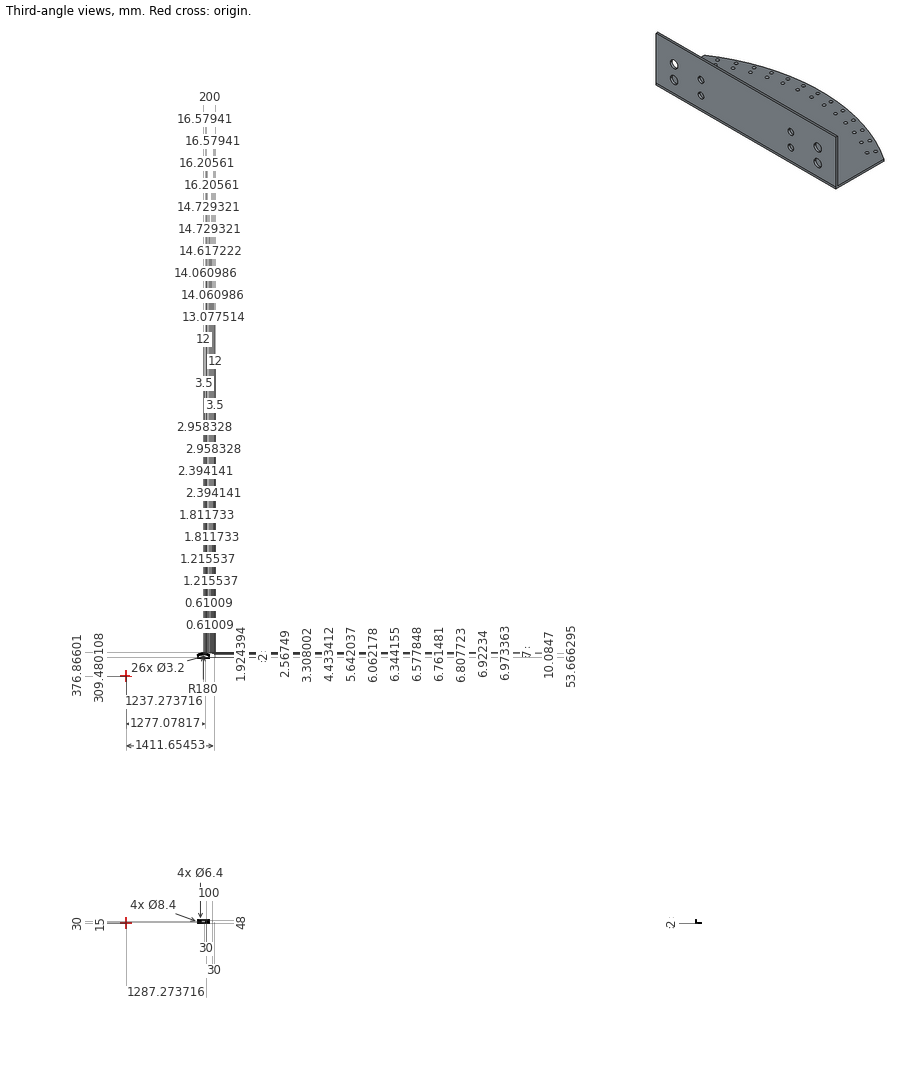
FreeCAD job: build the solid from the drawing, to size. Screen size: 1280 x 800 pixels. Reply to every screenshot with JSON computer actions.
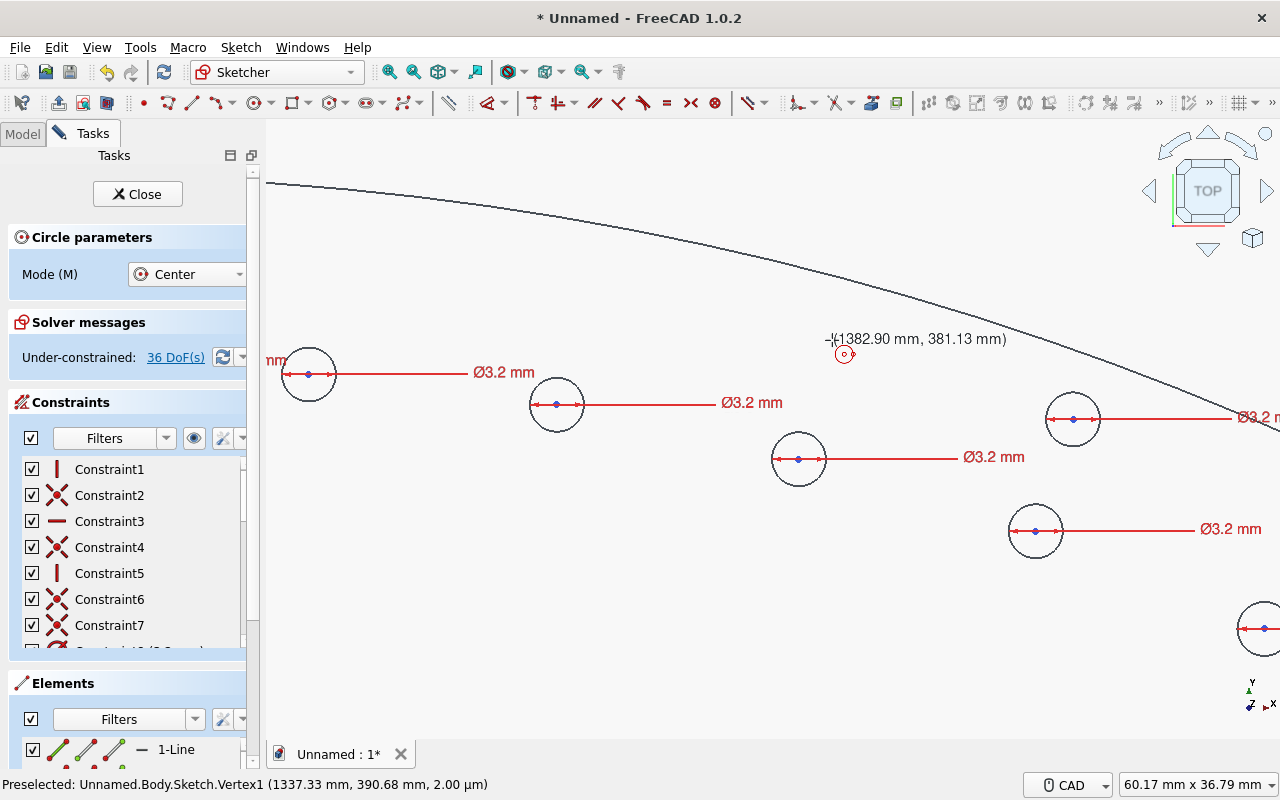
{"action": "scroll", "coordinate": [832, 340], "scroll_direction": "down", "scroll_amount": 9}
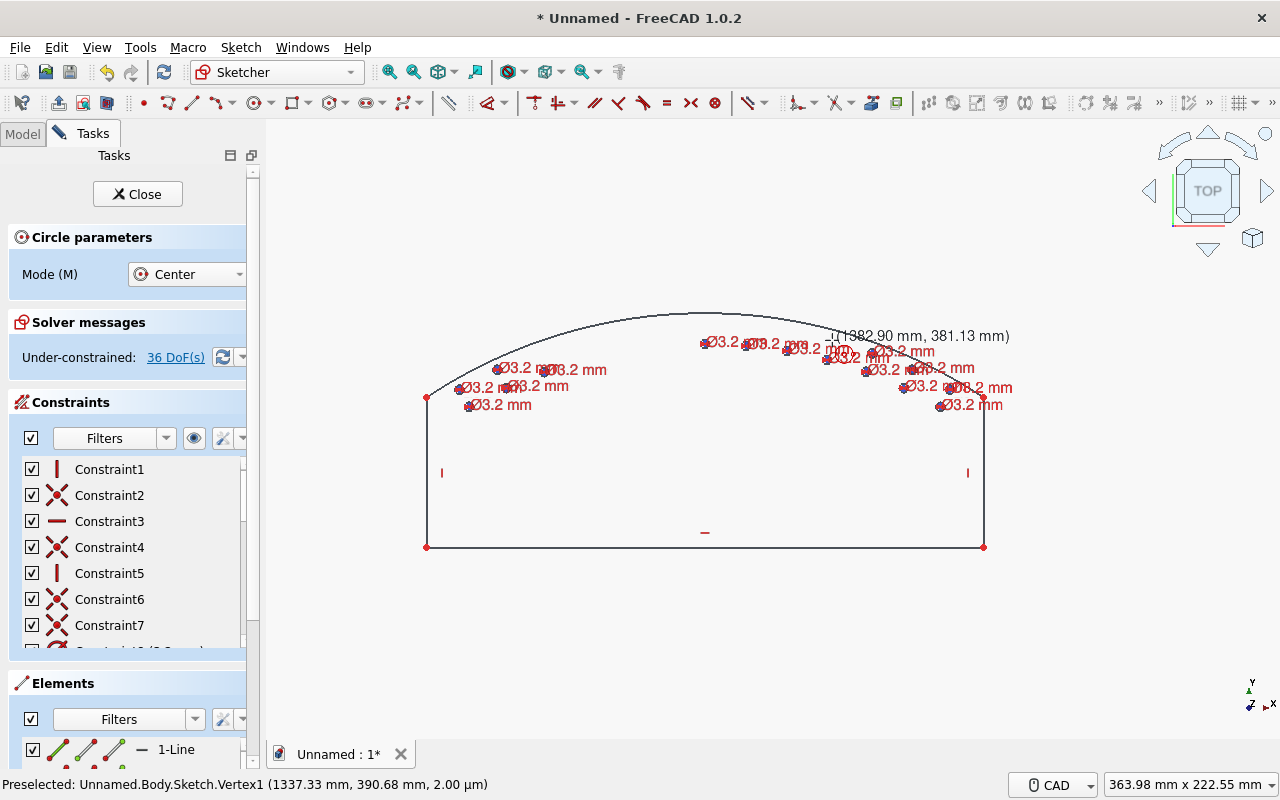
{"action": "scroll", "coordinate": [832, 340], "scroll_direction": "up", "scroll_amount": 2}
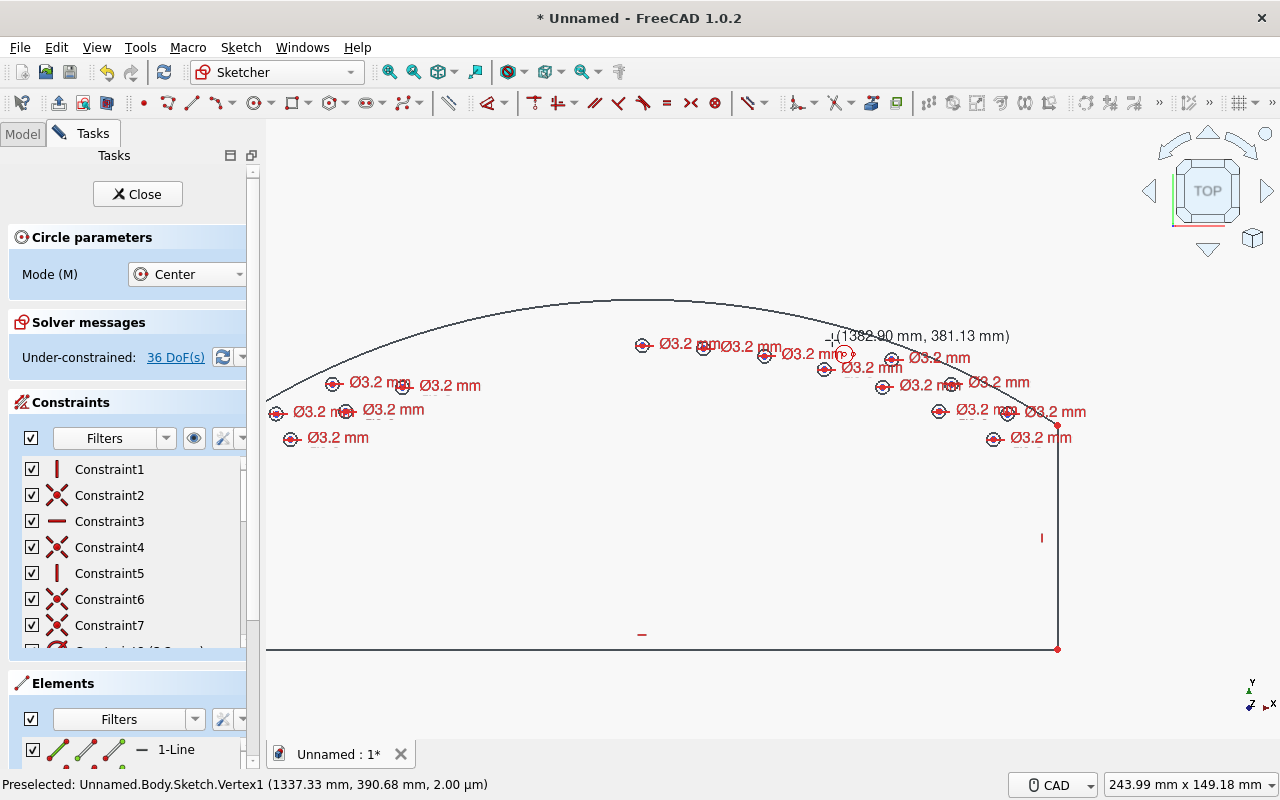
{"action": "left_click", "coordinate": [831, 340]}
{"action": "mouse_move", "coordinate": [836, 345]}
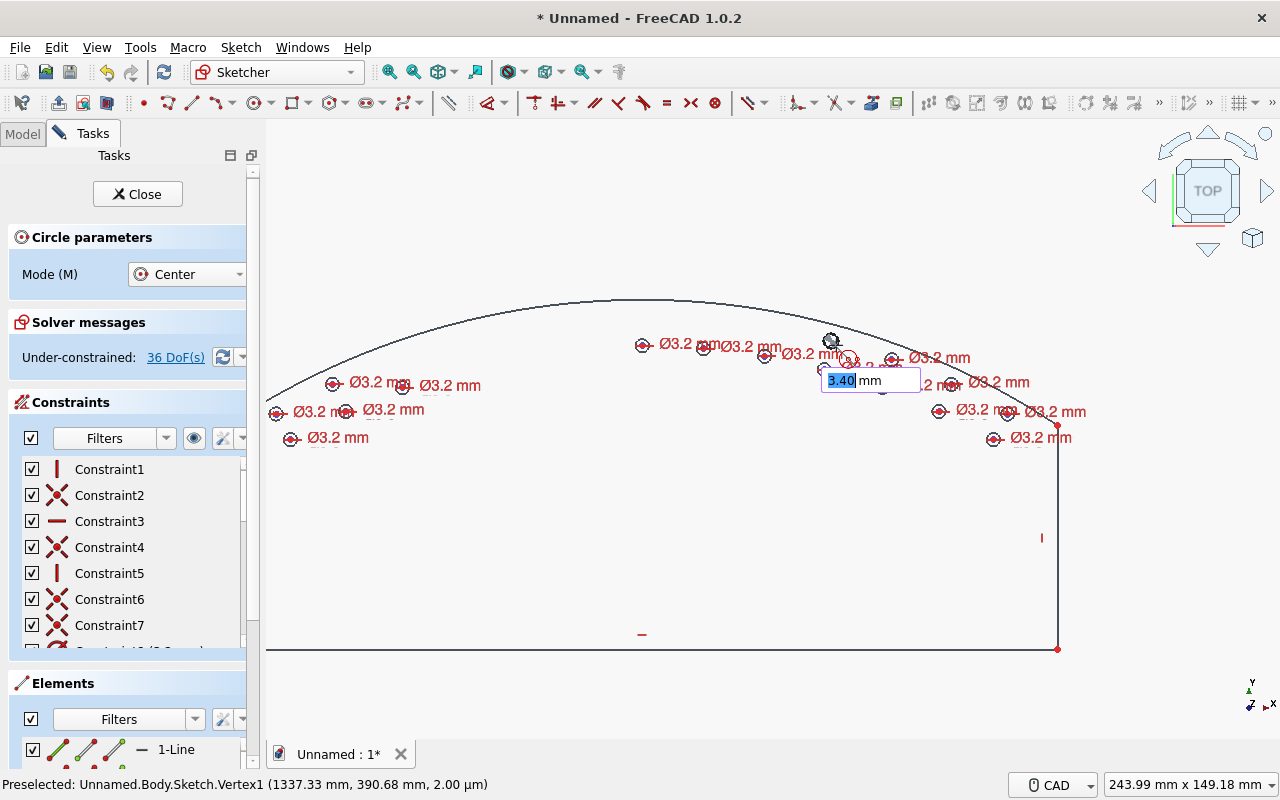
{"action": "type", "text": "3.2"}
{"action": "key", "text": "Return"}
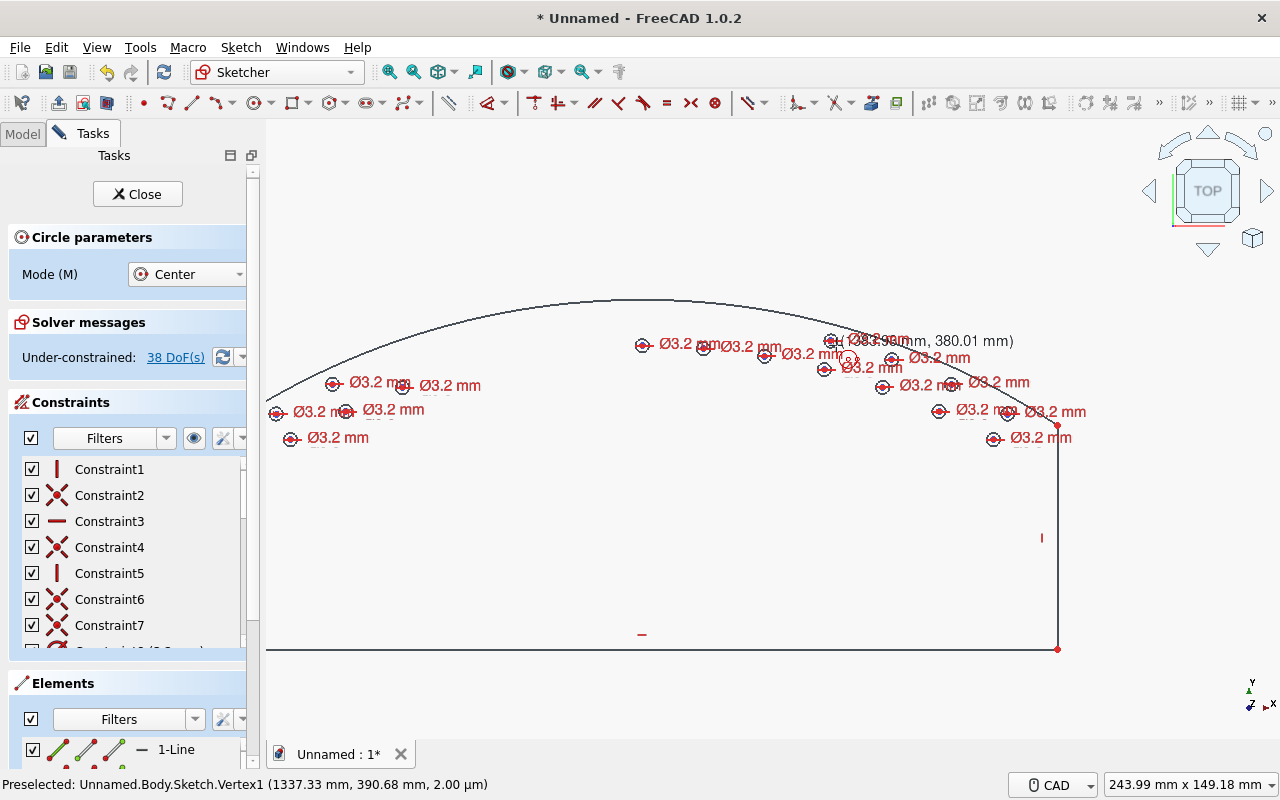
{"action": "scroll", "coordinate": [769, 326], "scroll_direction": "up", "scroll_amount": 7}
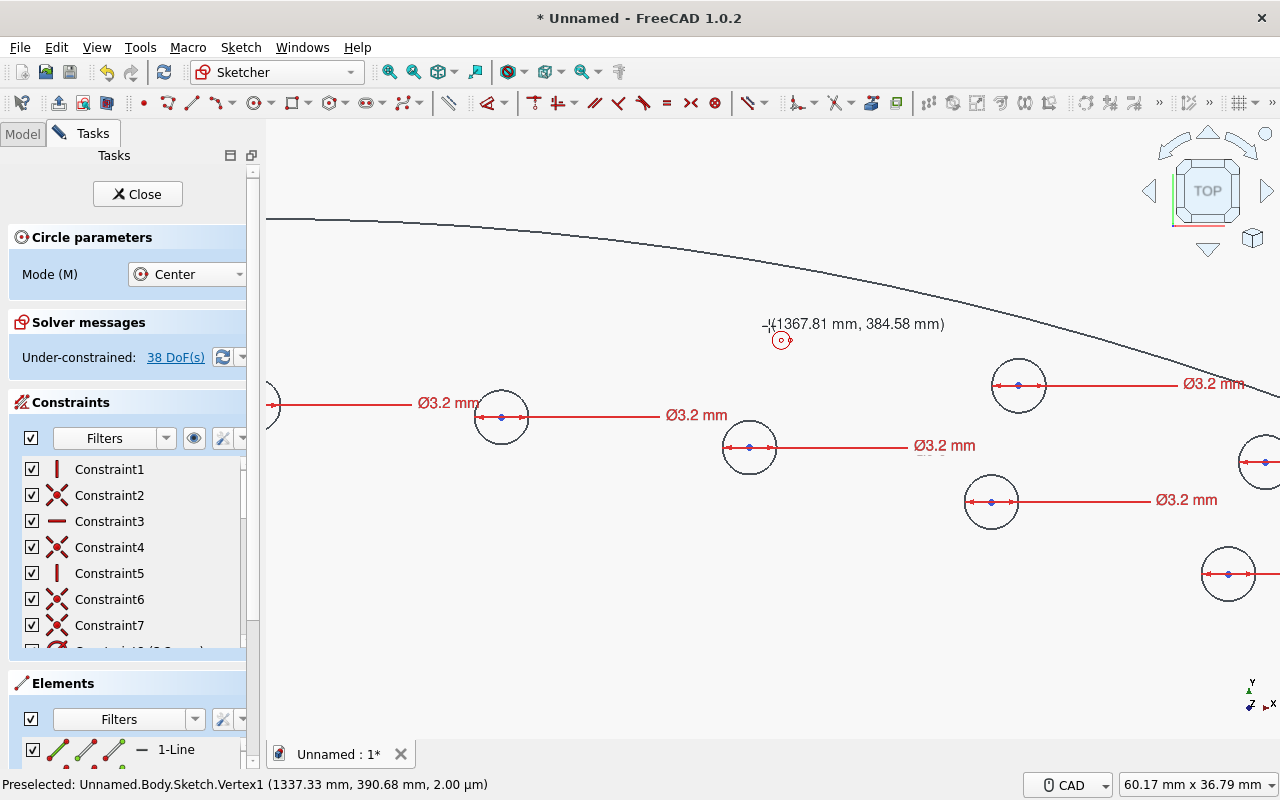
{"action": "scroll", "coordinate": [794, 332], "scroll_direction": "down", "scroll_amount": 9}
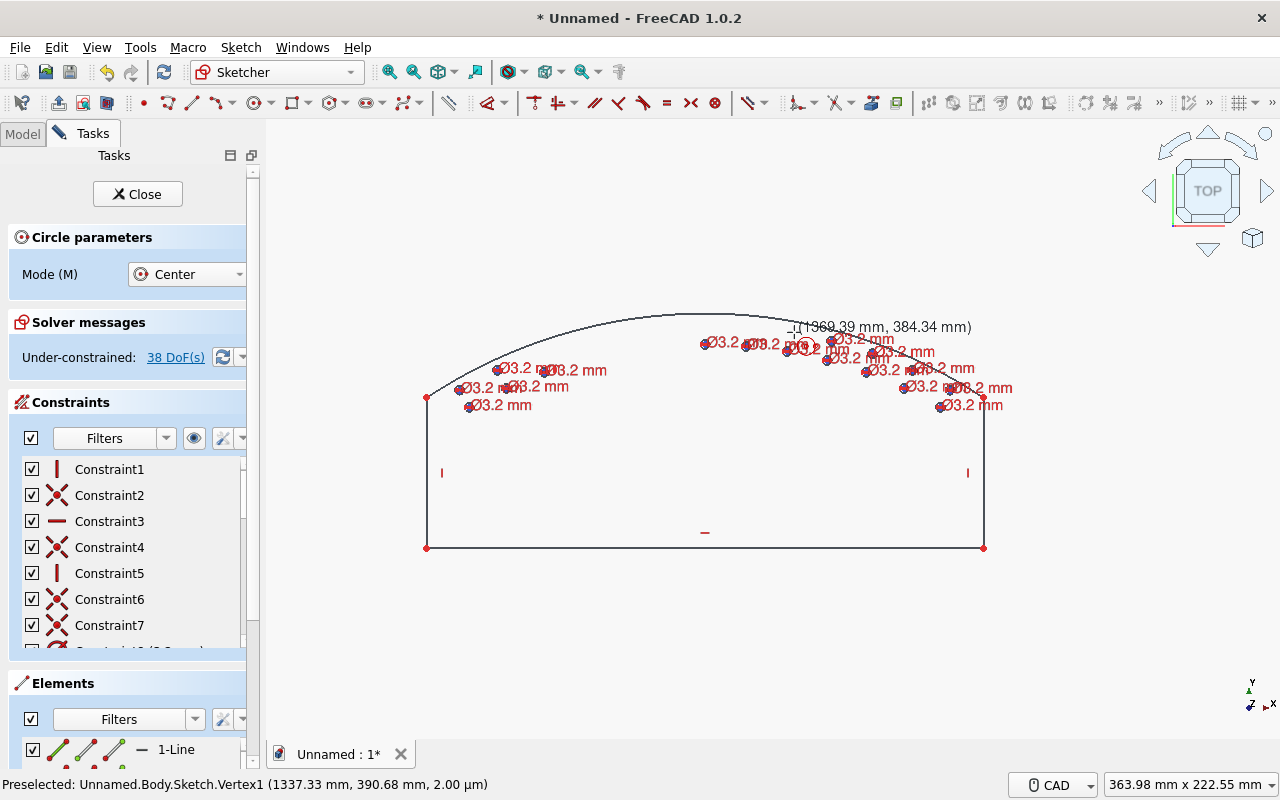
{"action": "scroll", "coordinate": [790, 331], "scroll_direction": "up", "scroll_amount": 2}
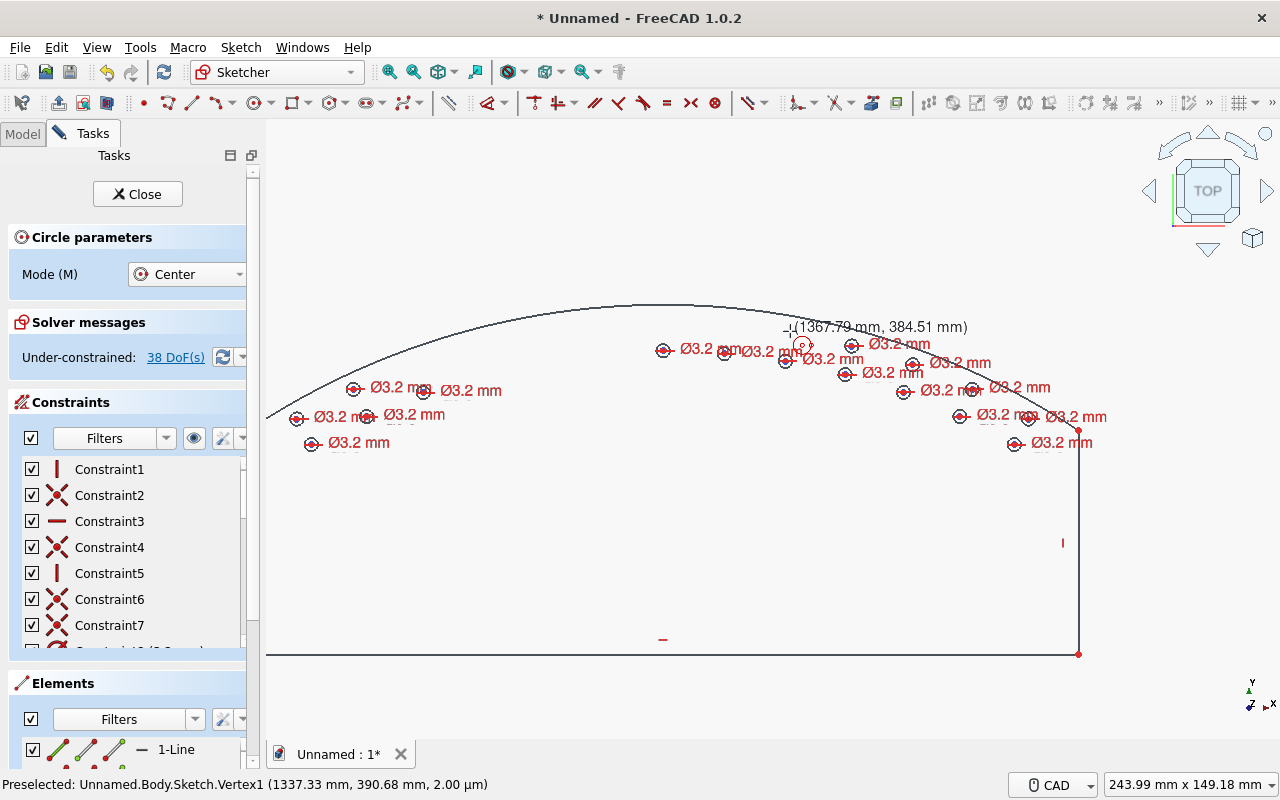
{"action": "left_click", "coordinate": [790, 331]}
{"action": "mouse_move", "coordinate": [795, 336]}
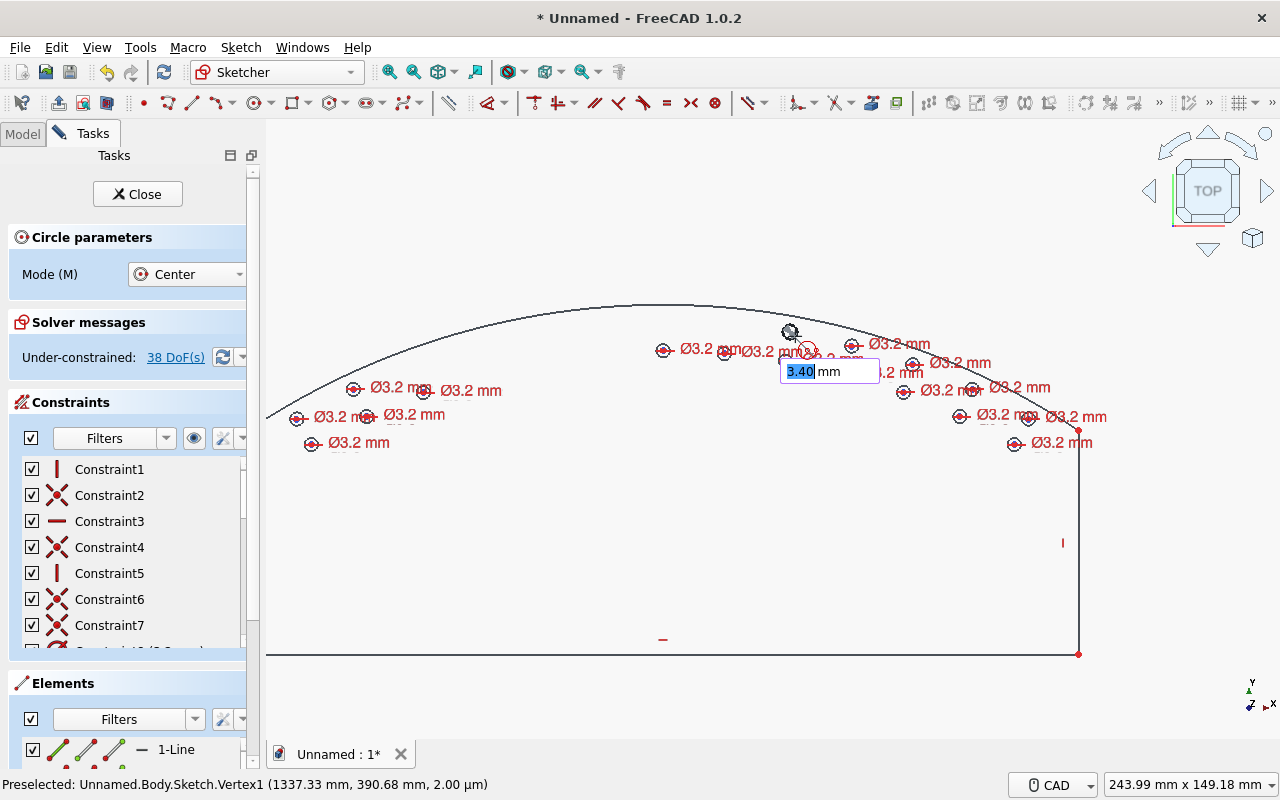
{"action": "type", "text": "3.2"}
{"action": "key", "text": "Return"}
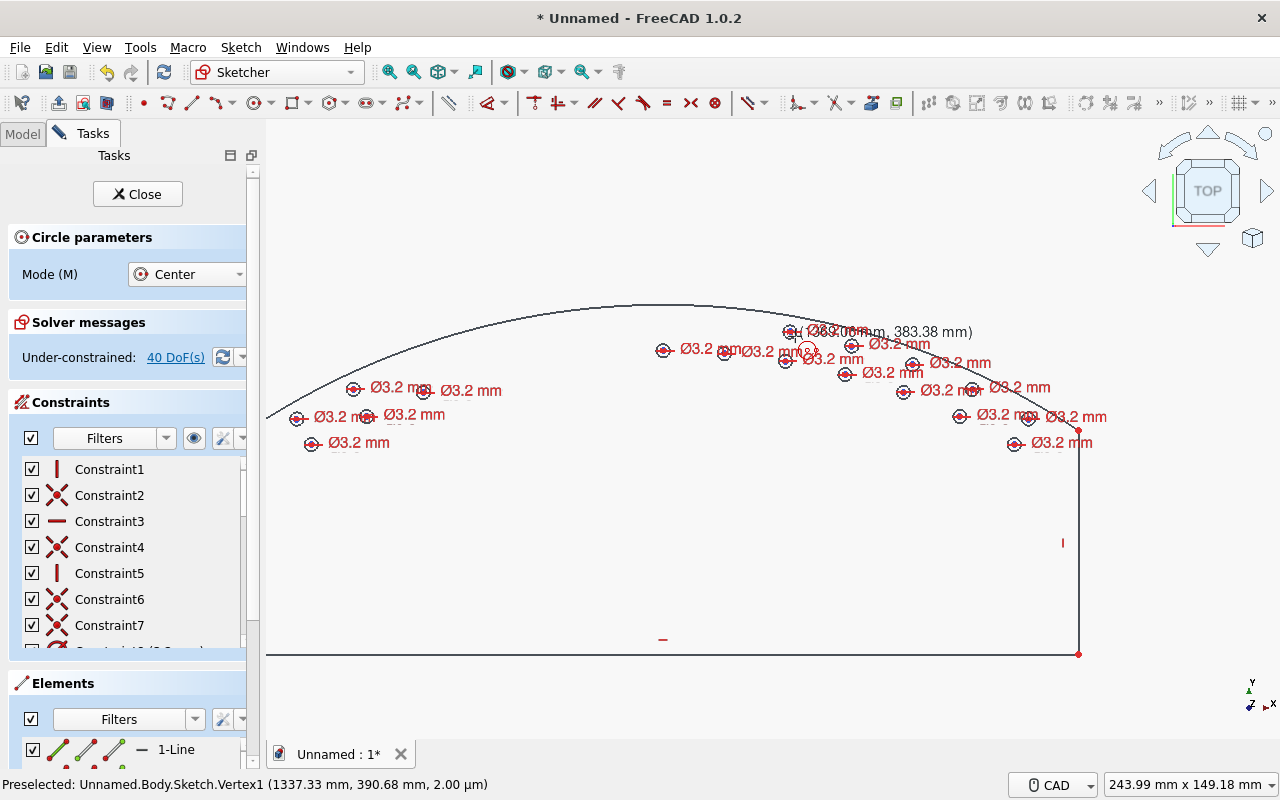
{"action": "scroll", "coordinate": [727, 323], "scroll_direction": "up", "scroll_amount": 7}